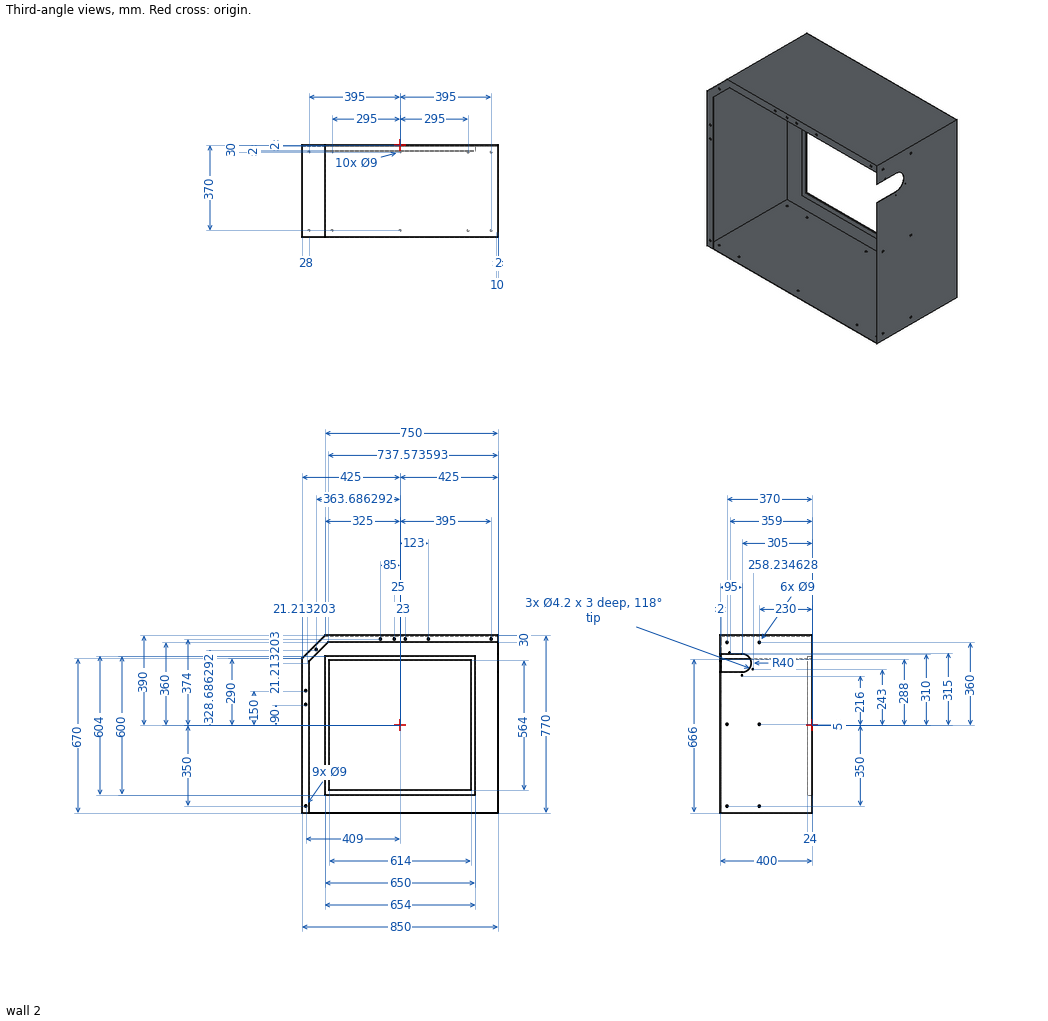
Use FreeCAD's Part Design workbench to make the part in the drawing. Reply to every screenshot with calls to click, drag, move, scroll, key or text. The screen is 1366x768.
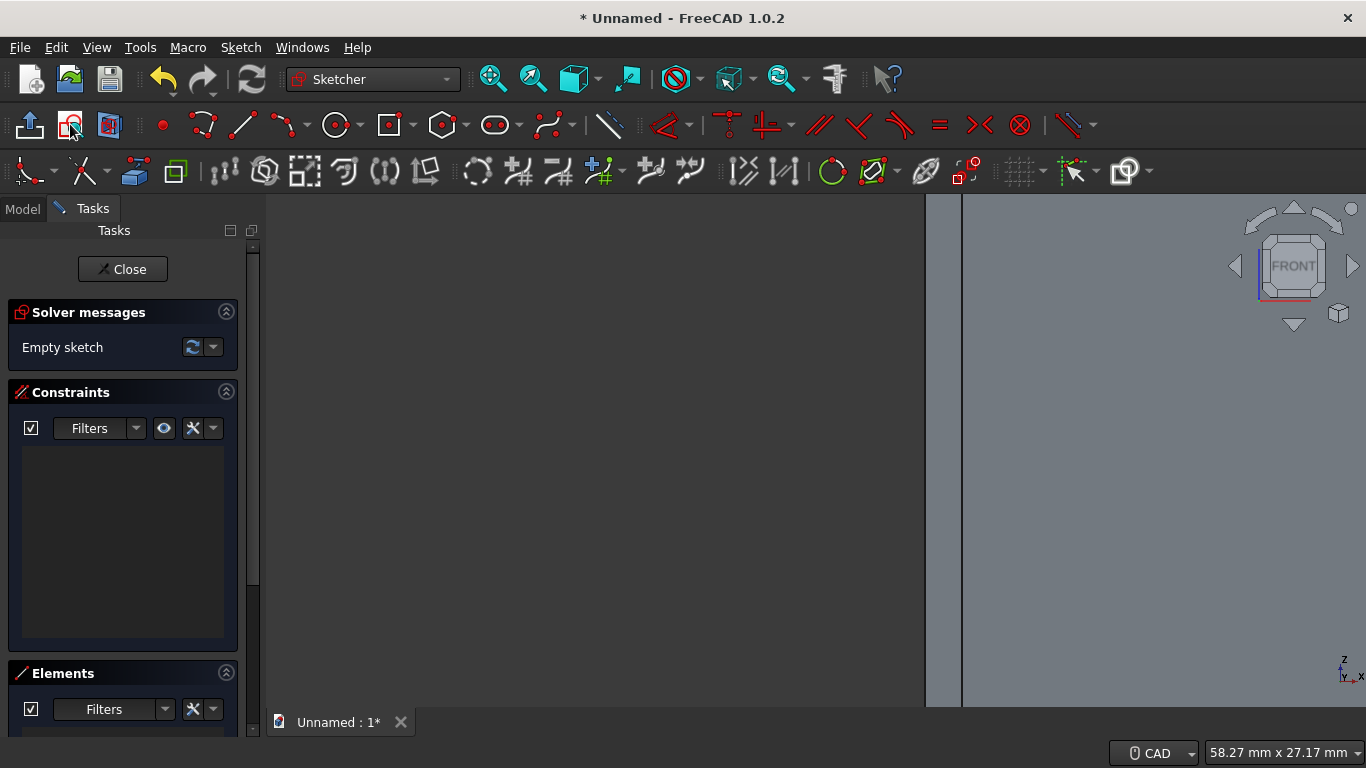
click(110, 126)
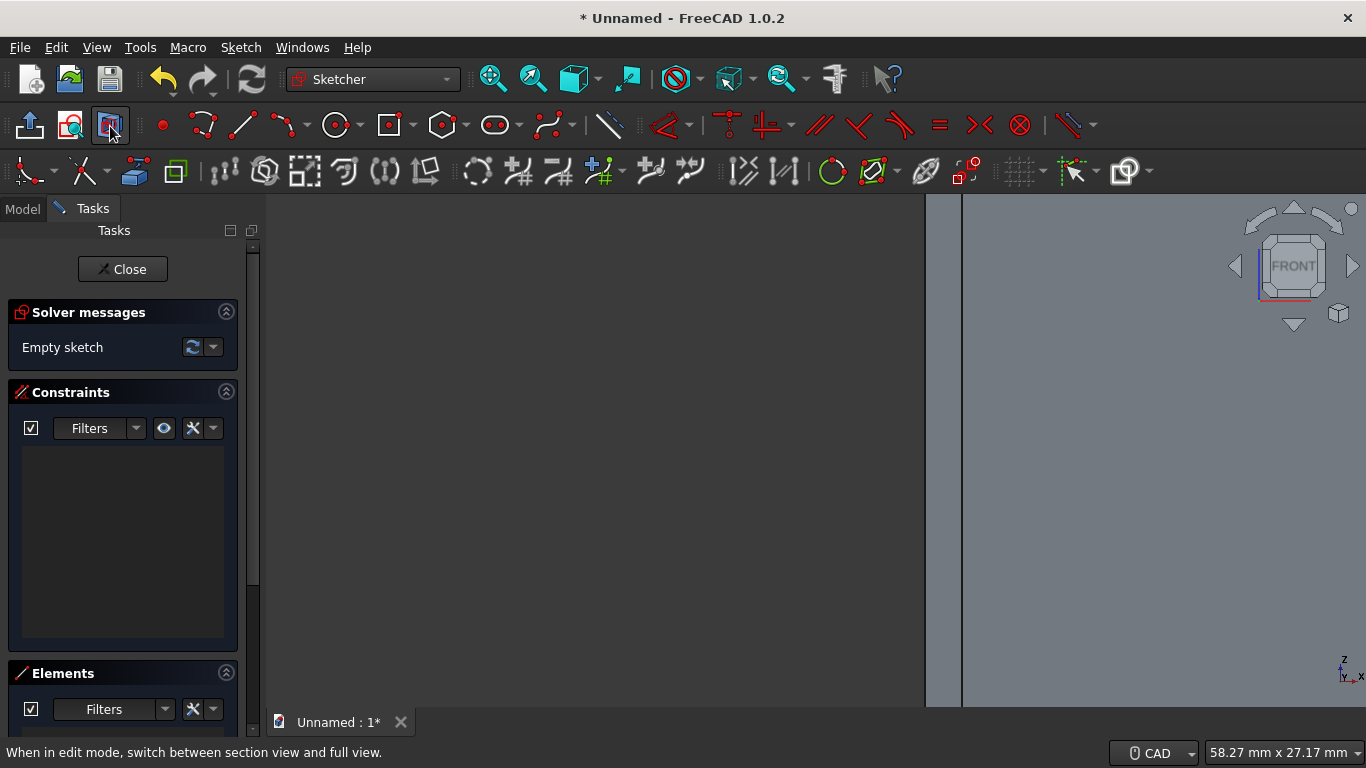
scroll(953, 514, down, 17)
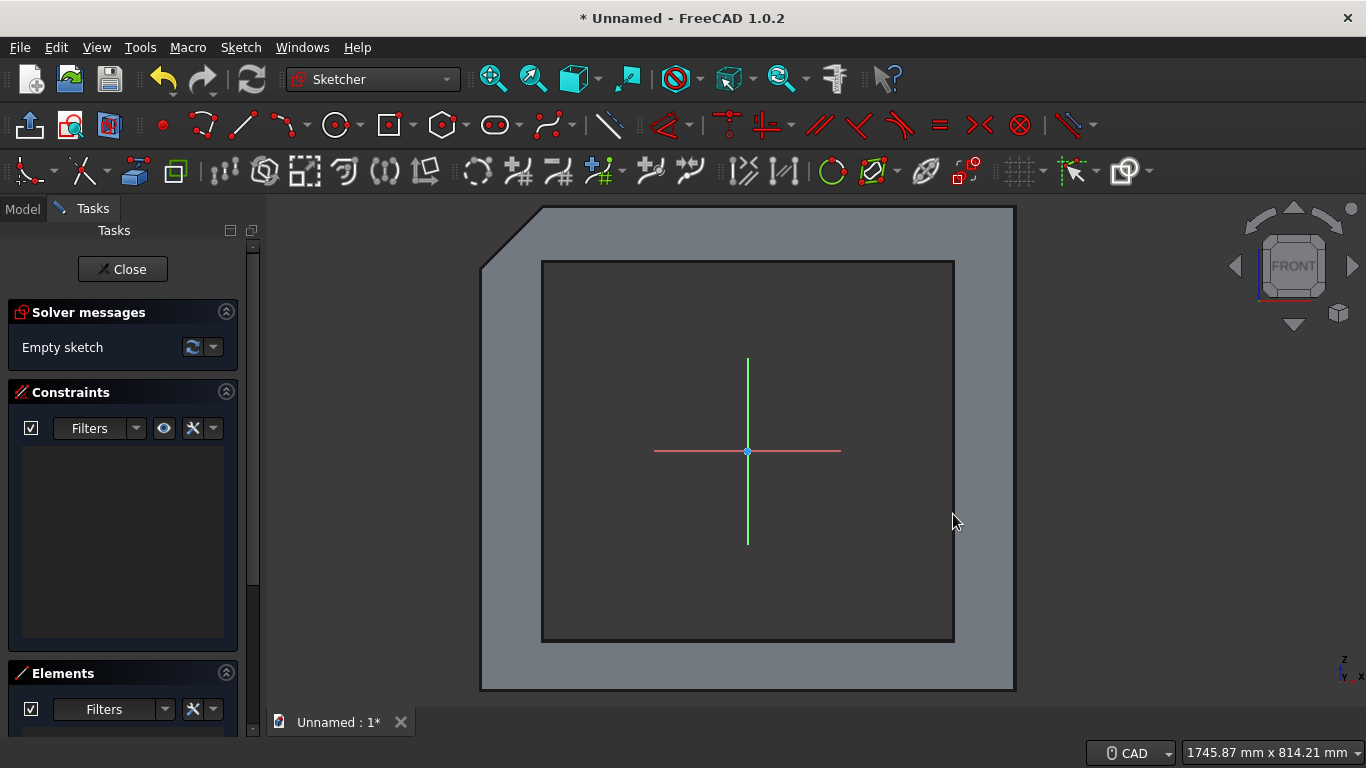
click(390, 126)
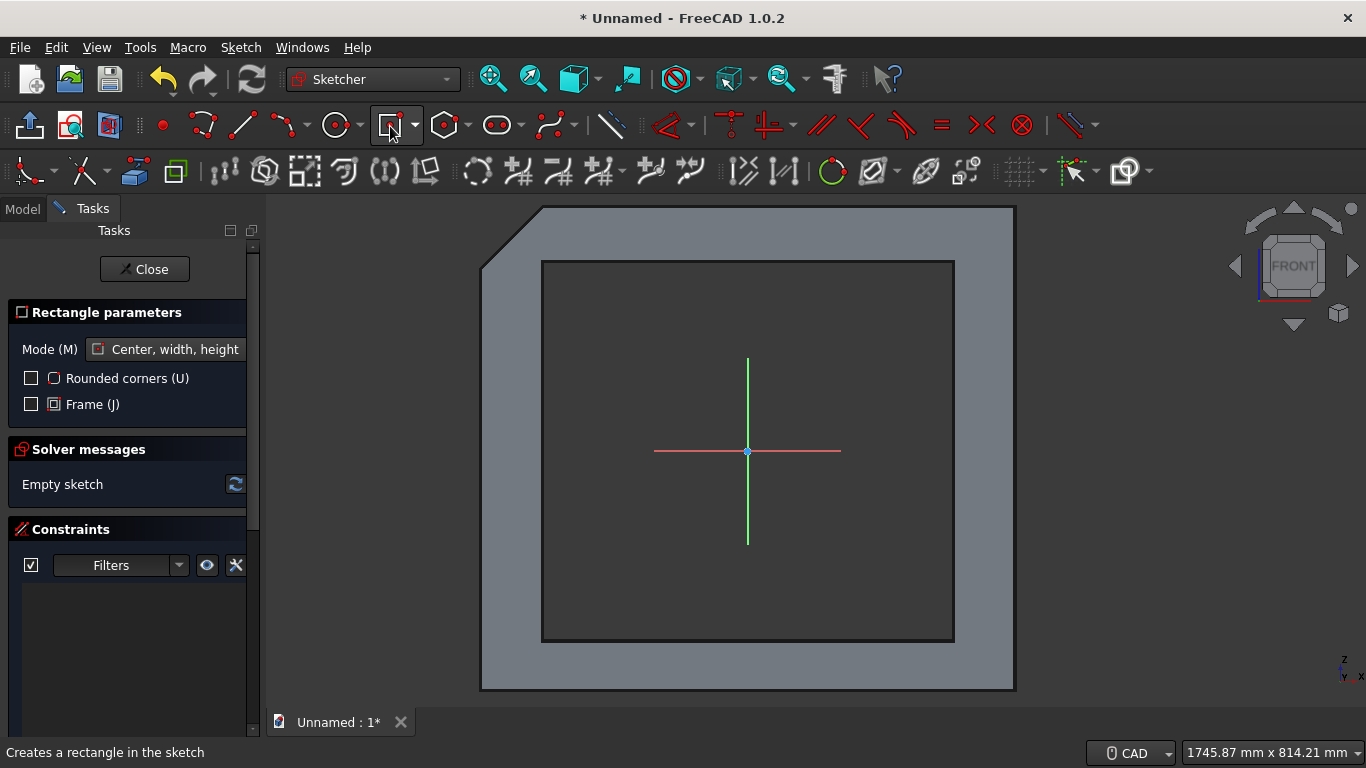
click(748, 451)
move(954, 261)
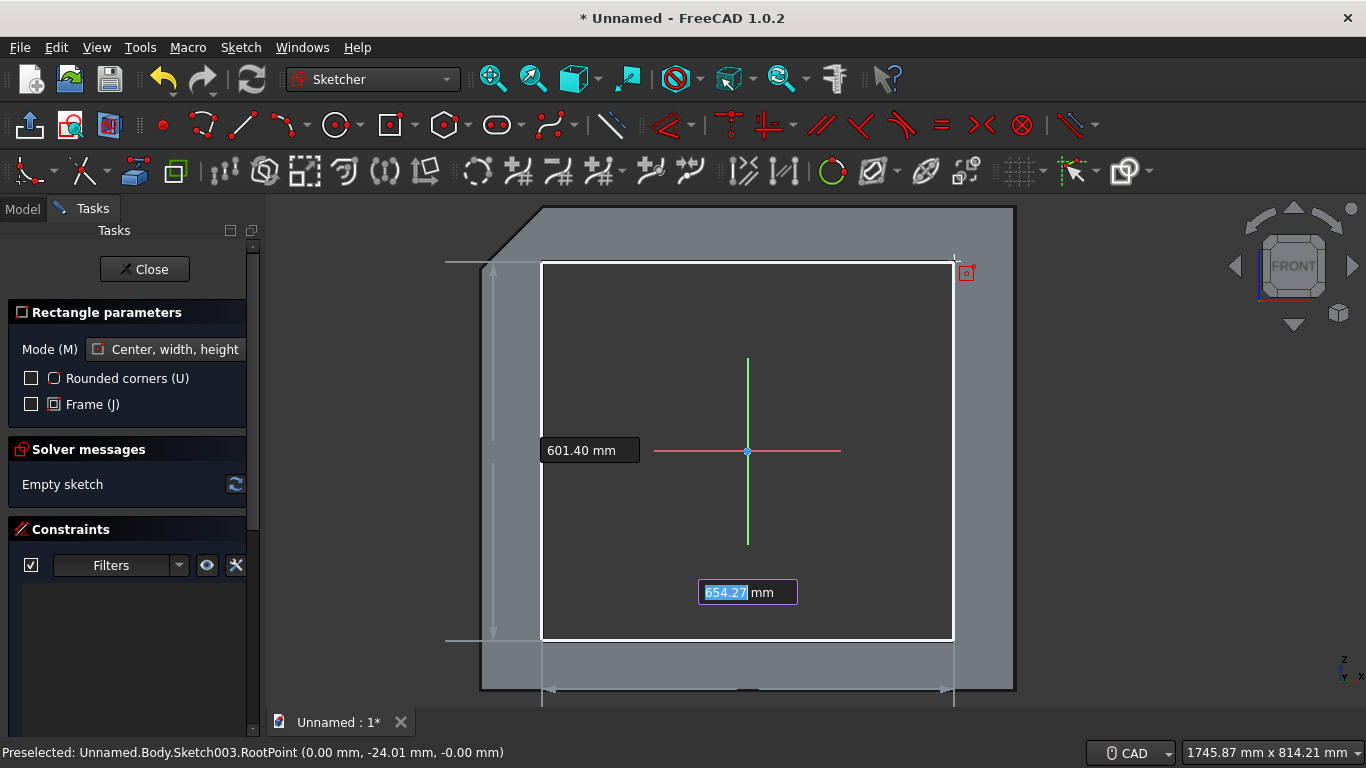
text(654)
key(Tab)
text(604)
key(Return)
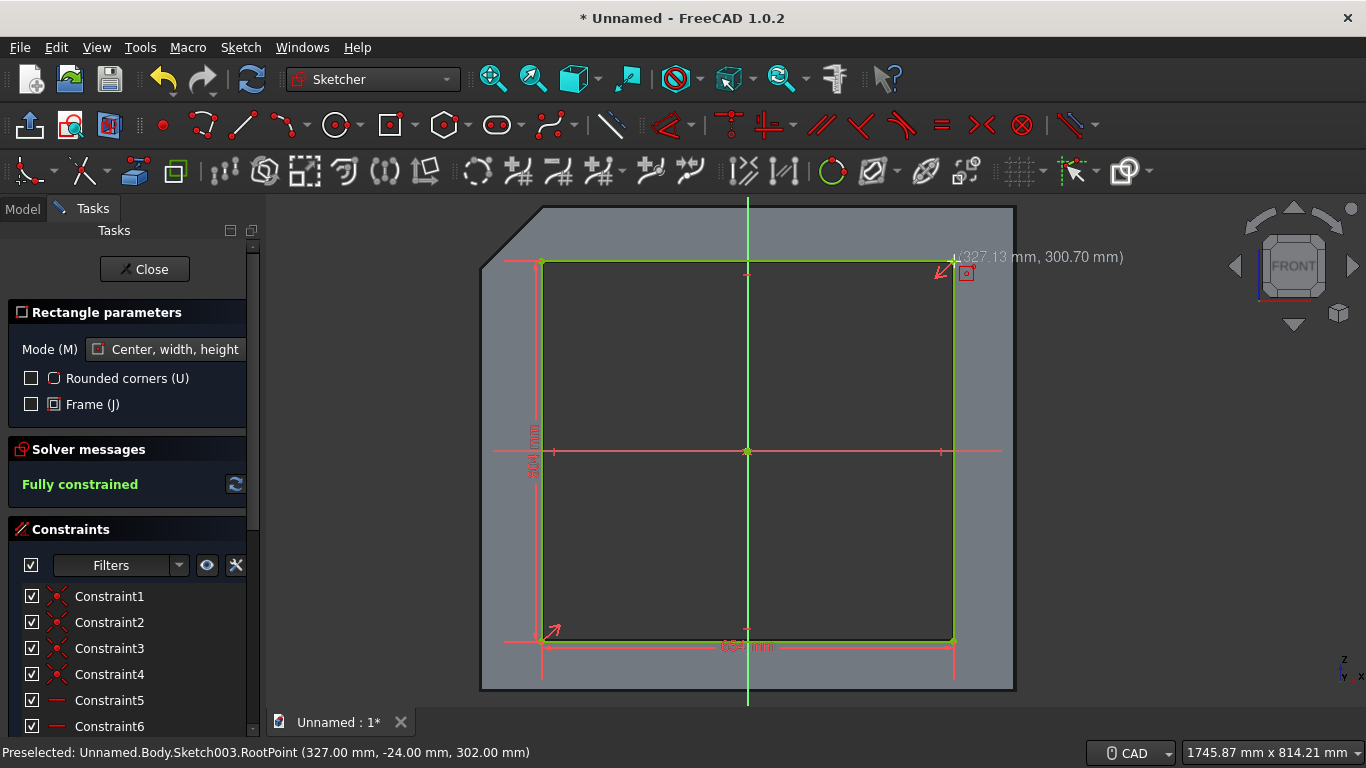
click(748, 451)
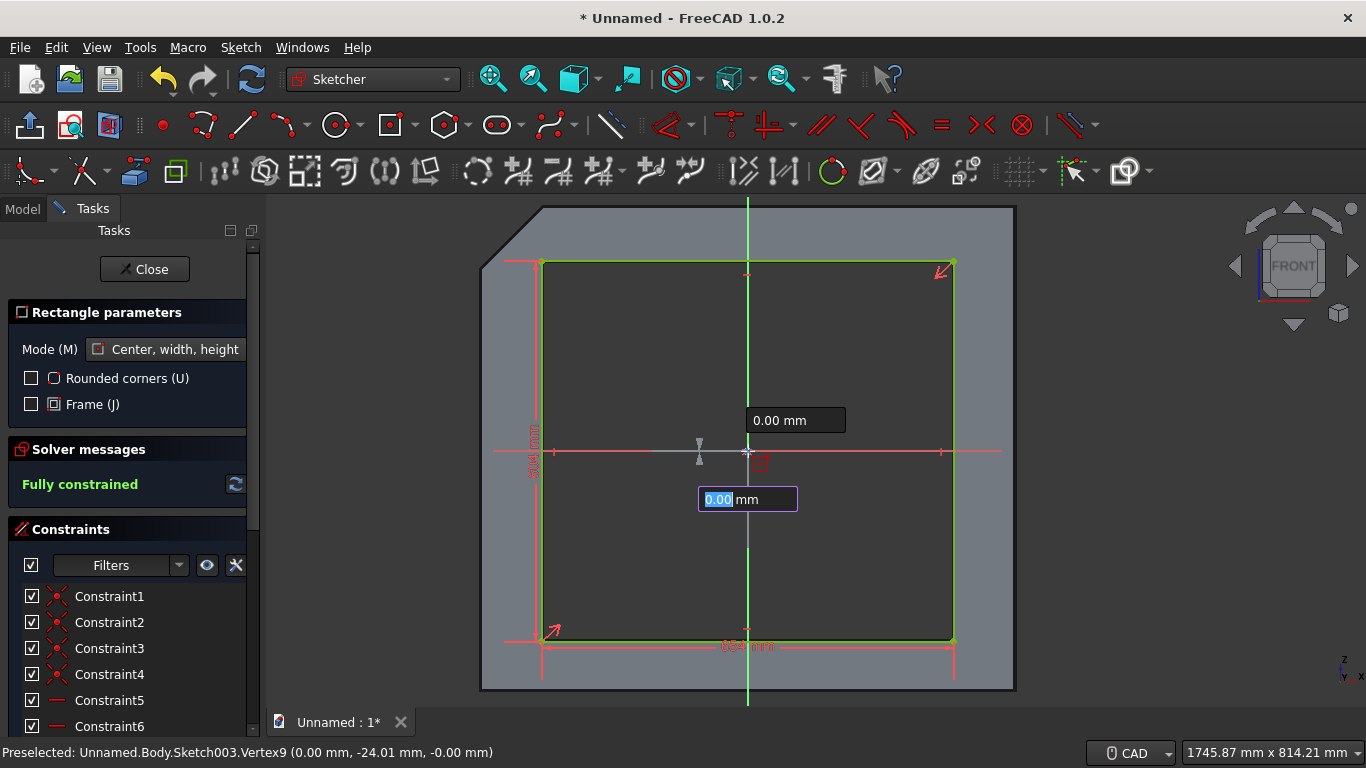
scroll(941, 274, up, 2)
move(941, 274)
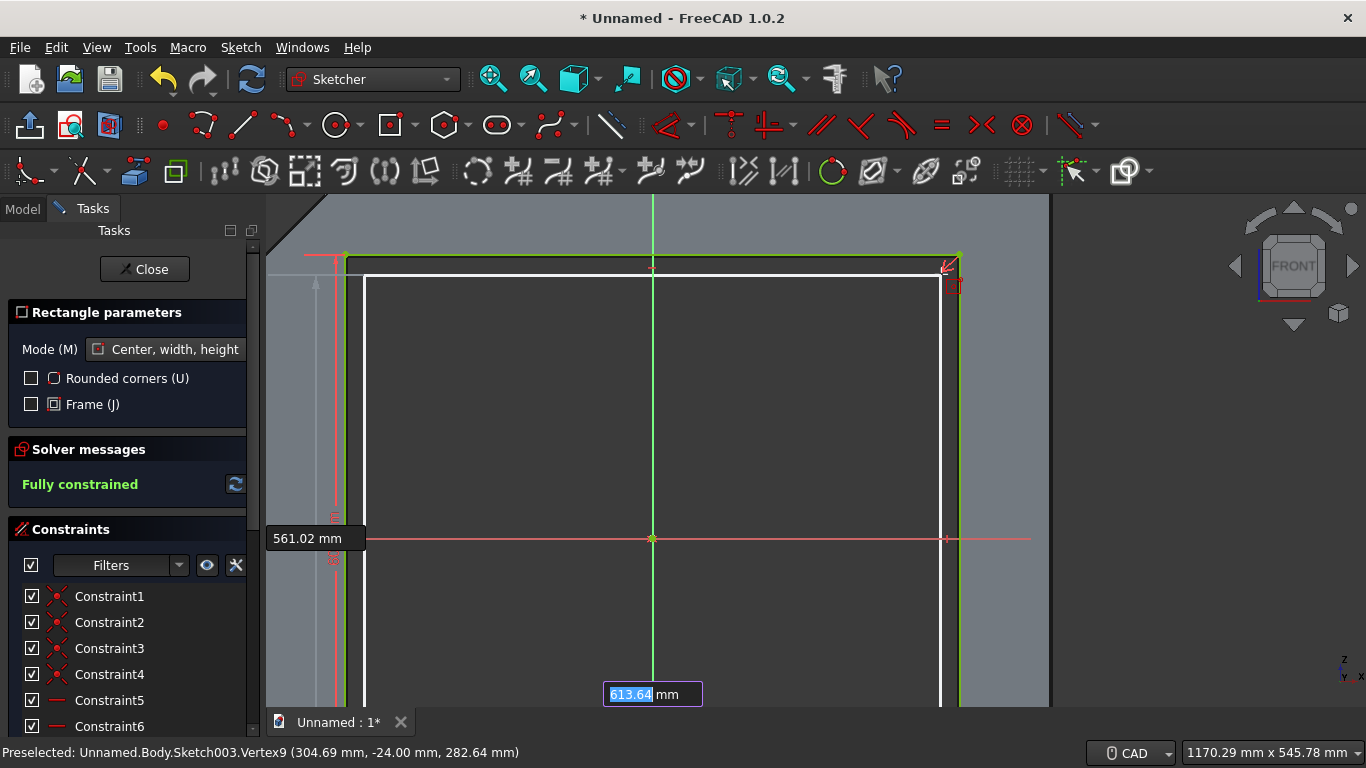
text(614)
key(Tab)
text(564)
key(Return)
key(Escape)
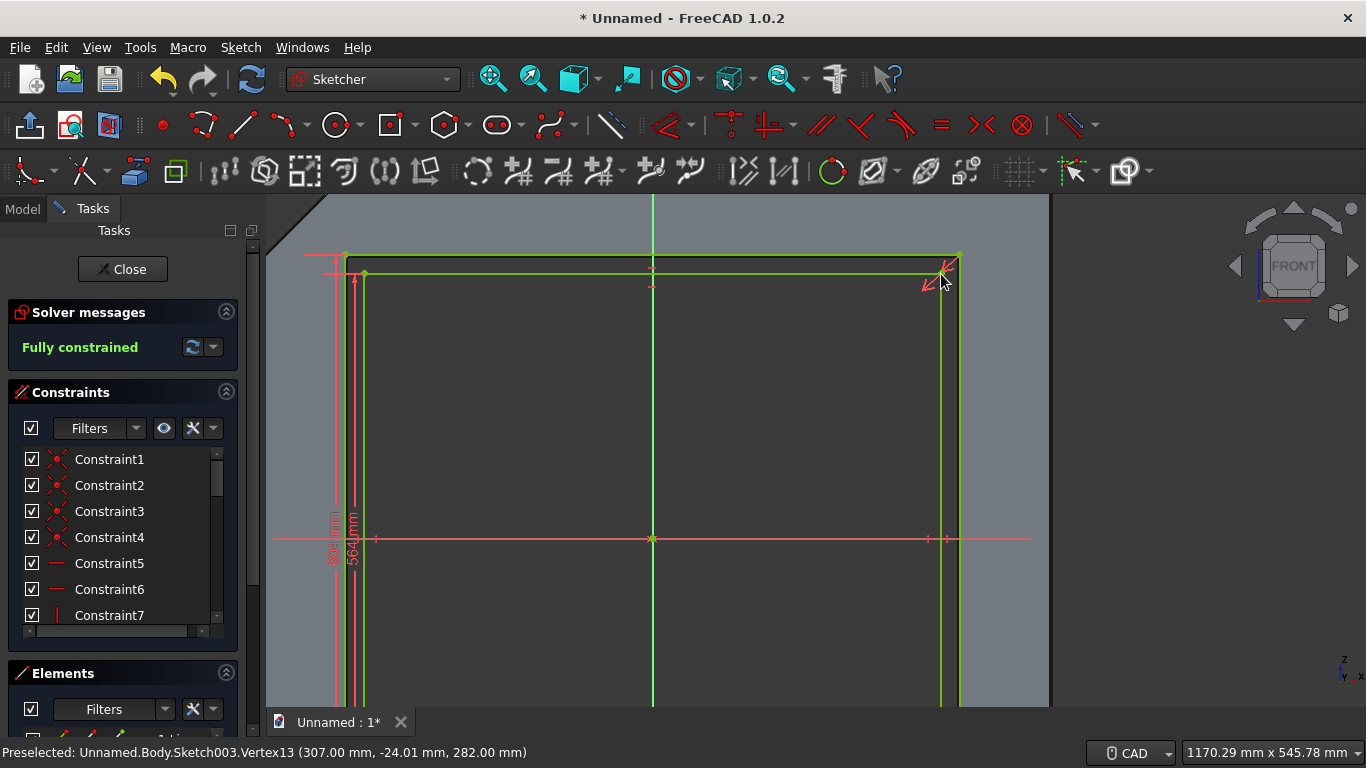
click(123, 269)